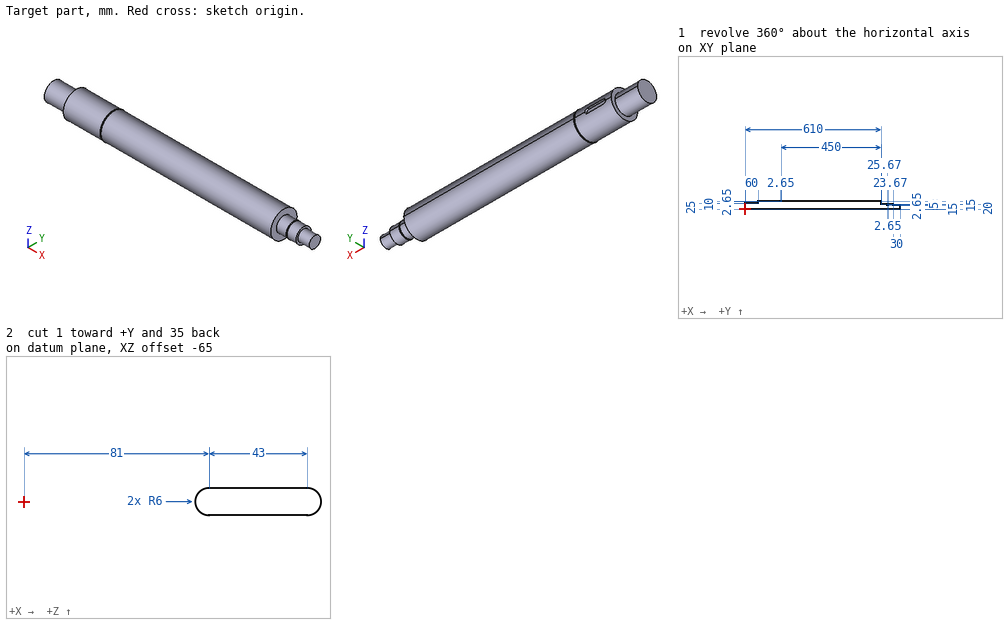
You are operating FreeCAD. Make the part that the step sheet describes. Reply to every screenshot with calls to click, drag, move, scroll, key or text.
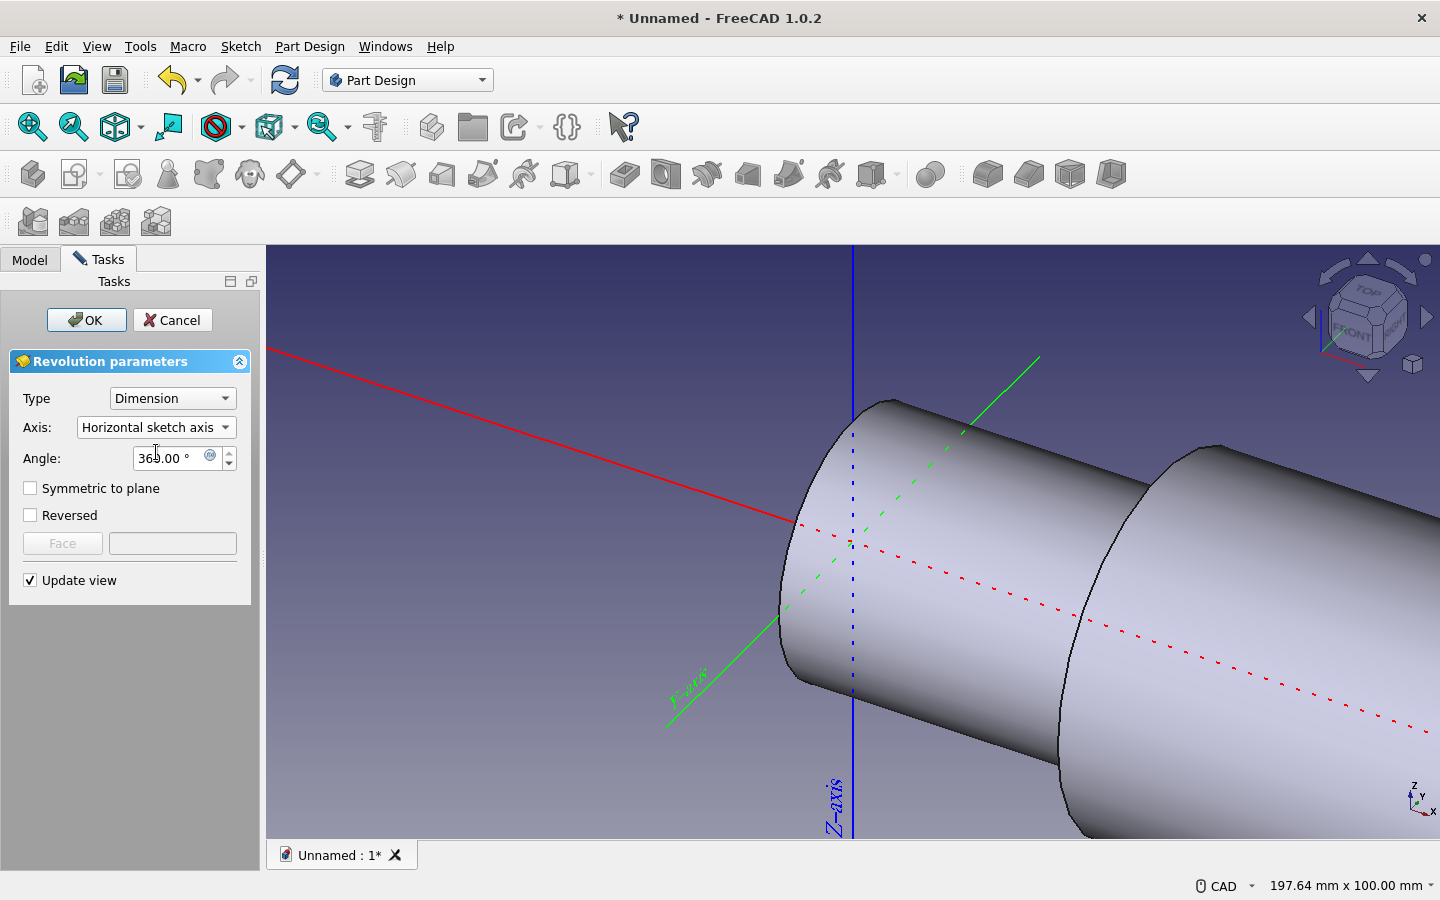
click(87, 320)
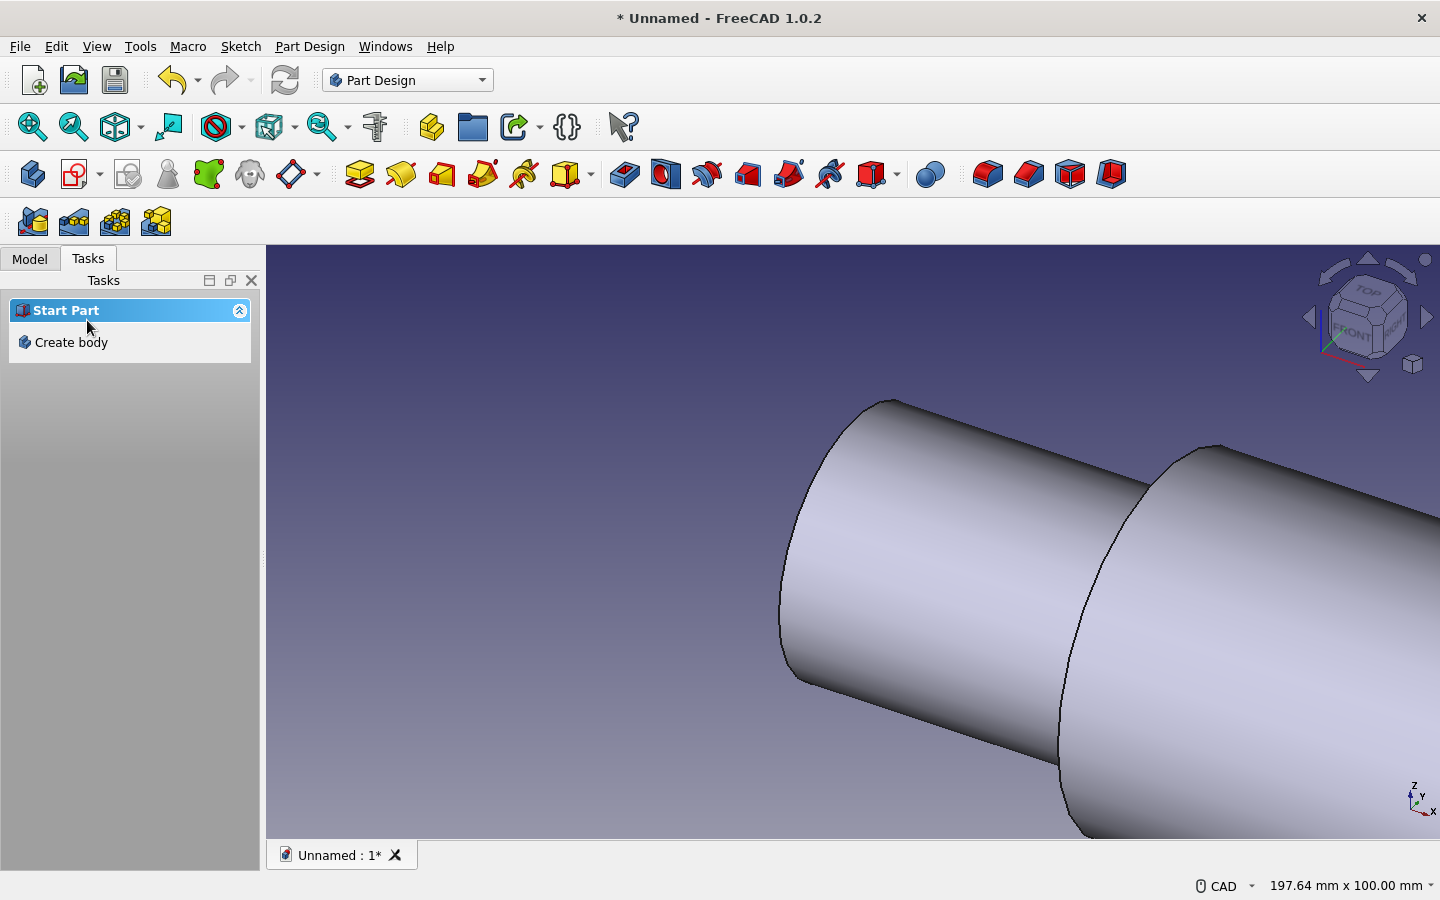
click(33, 128)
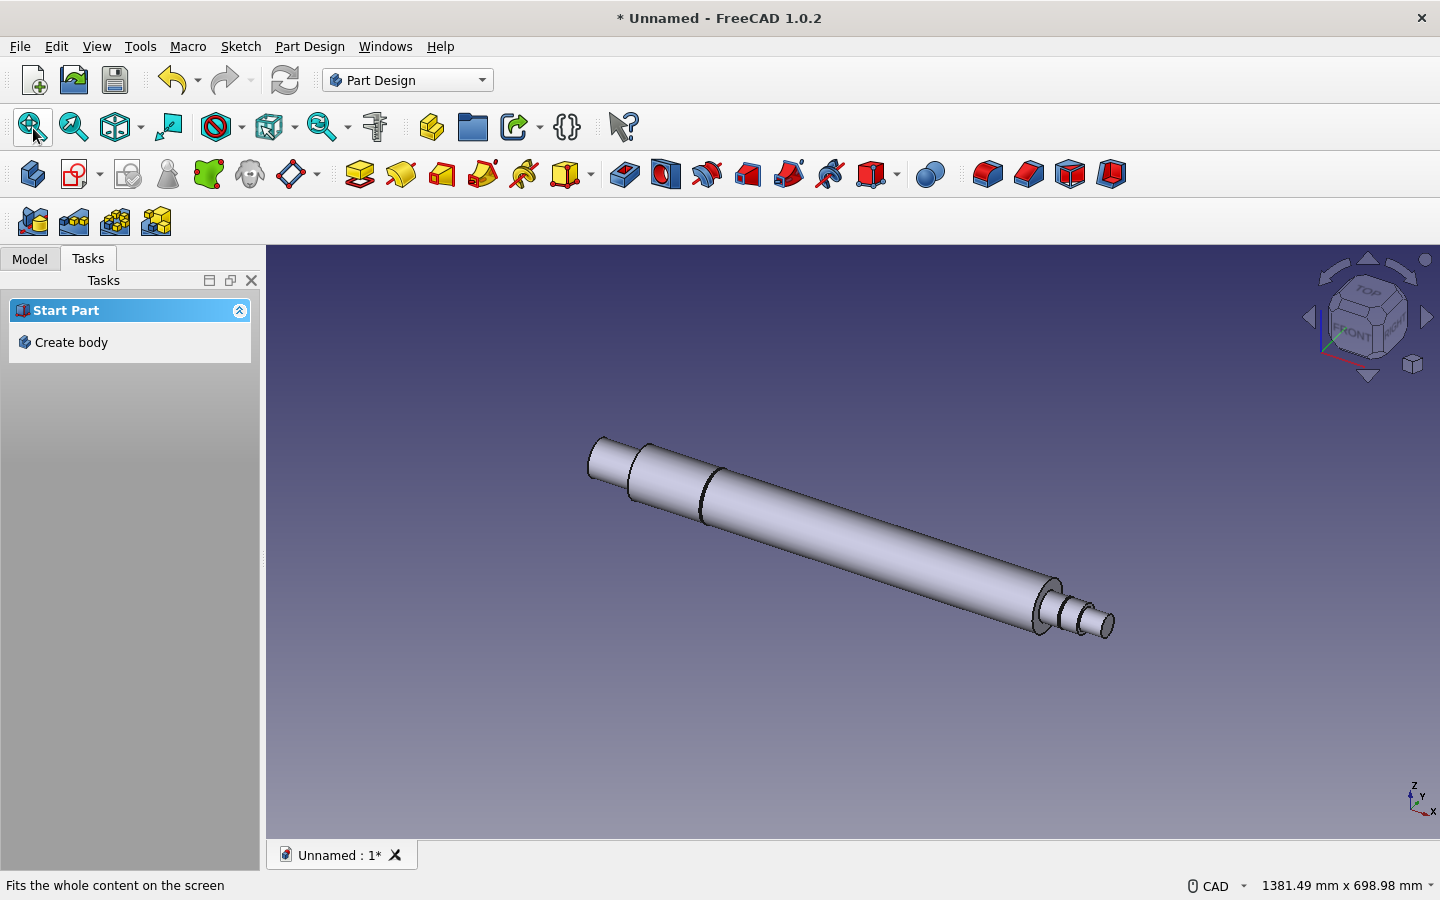
click(30, 258)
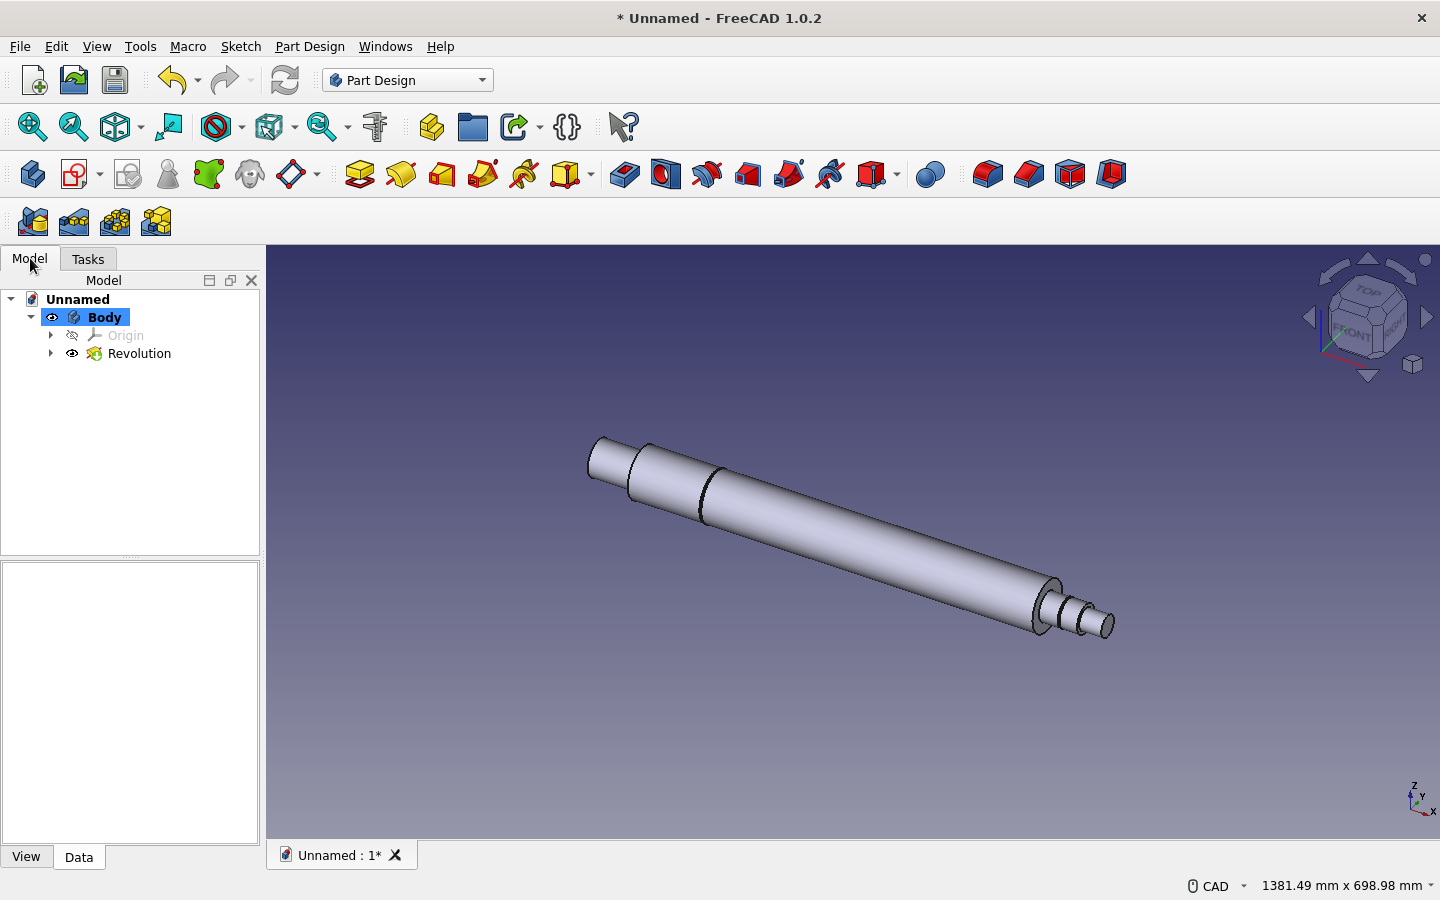
click(51, 335)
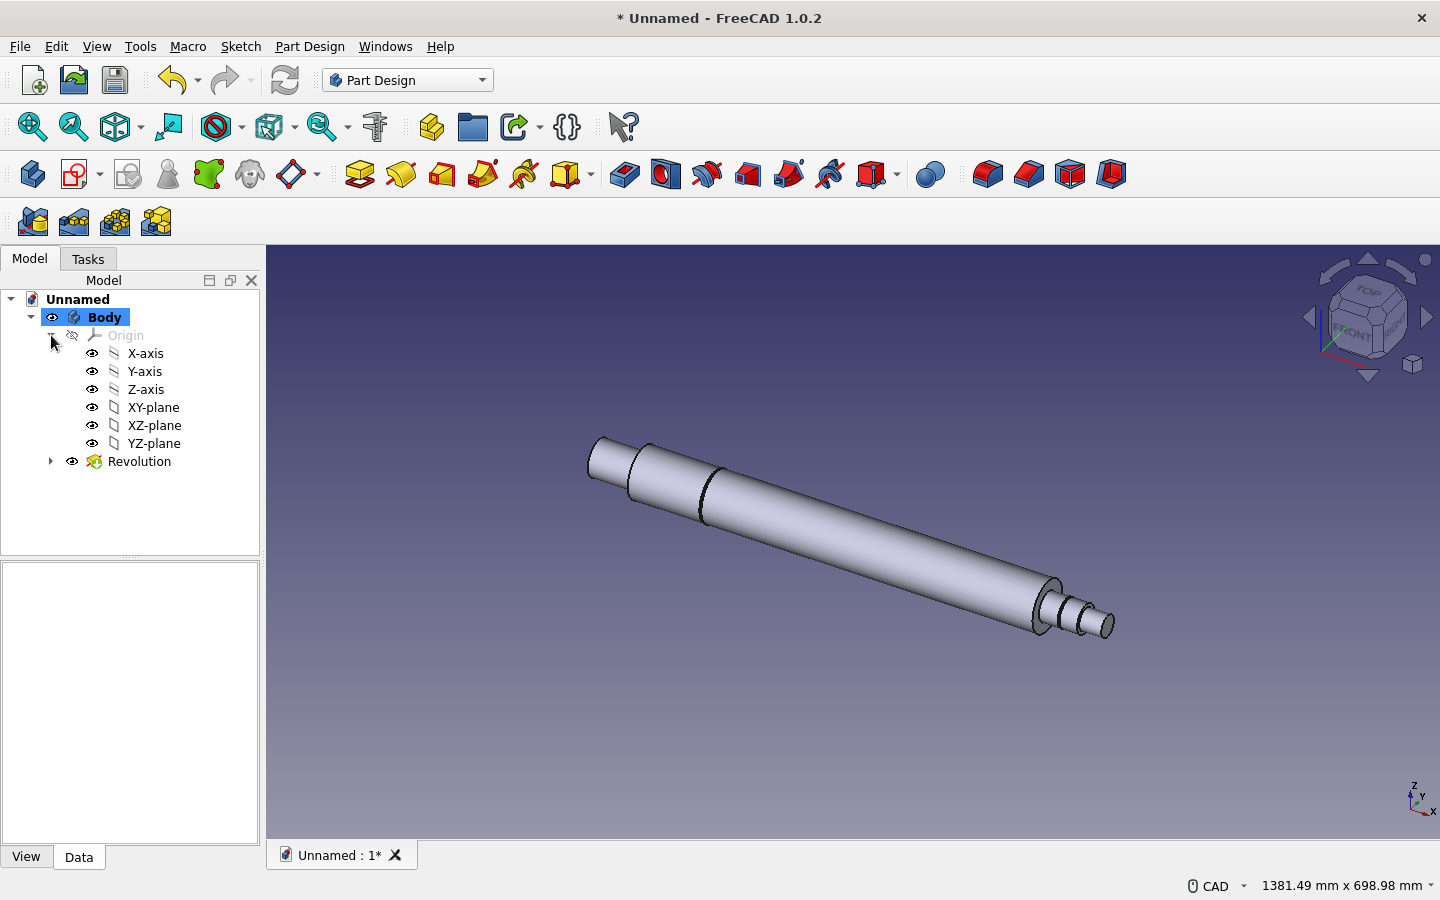
click(137, 425)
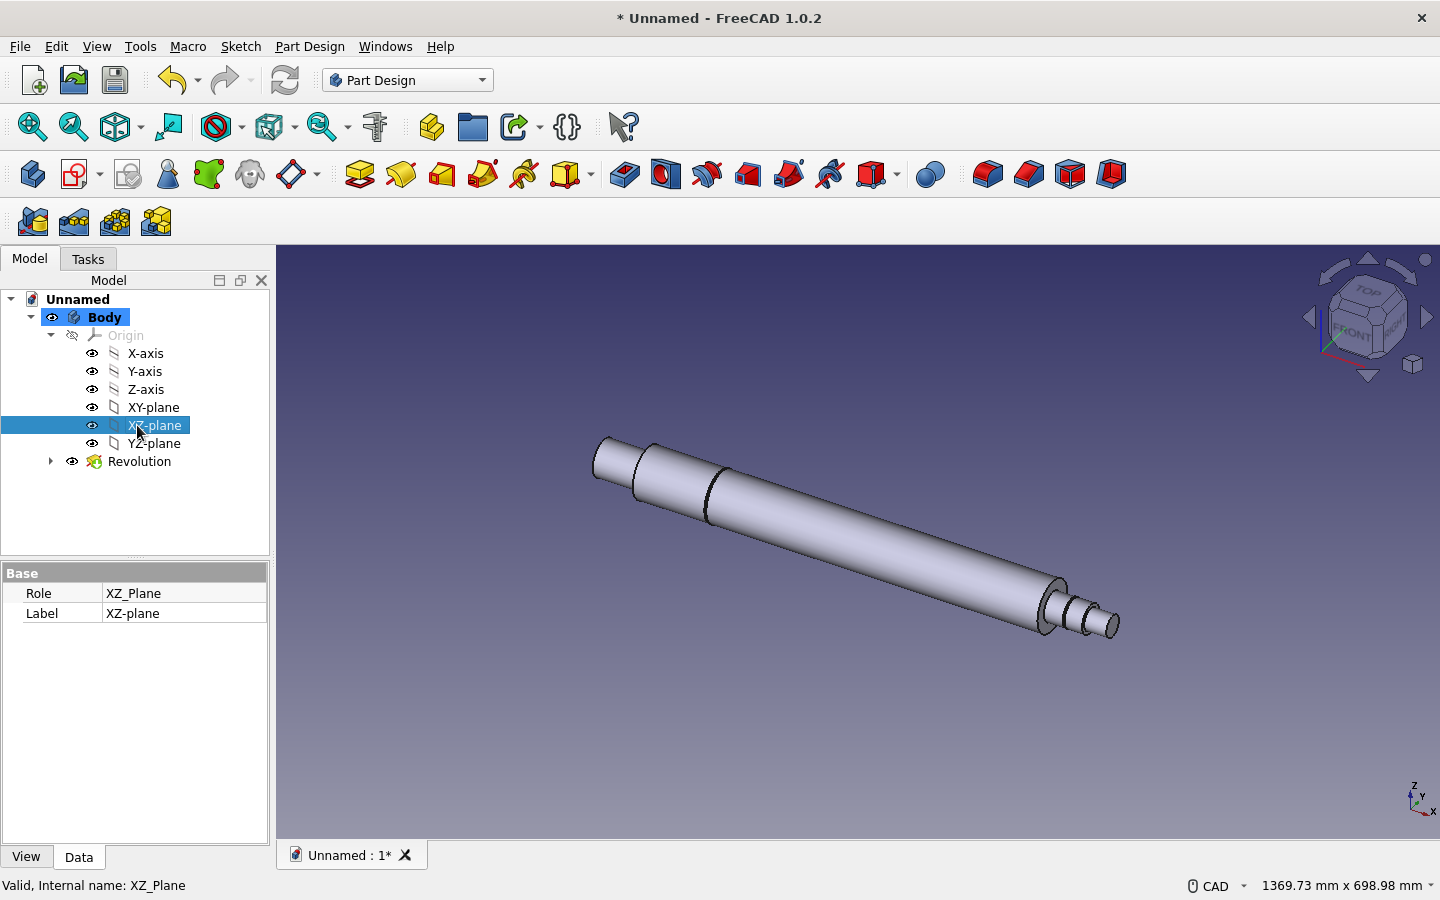
click(290, 174)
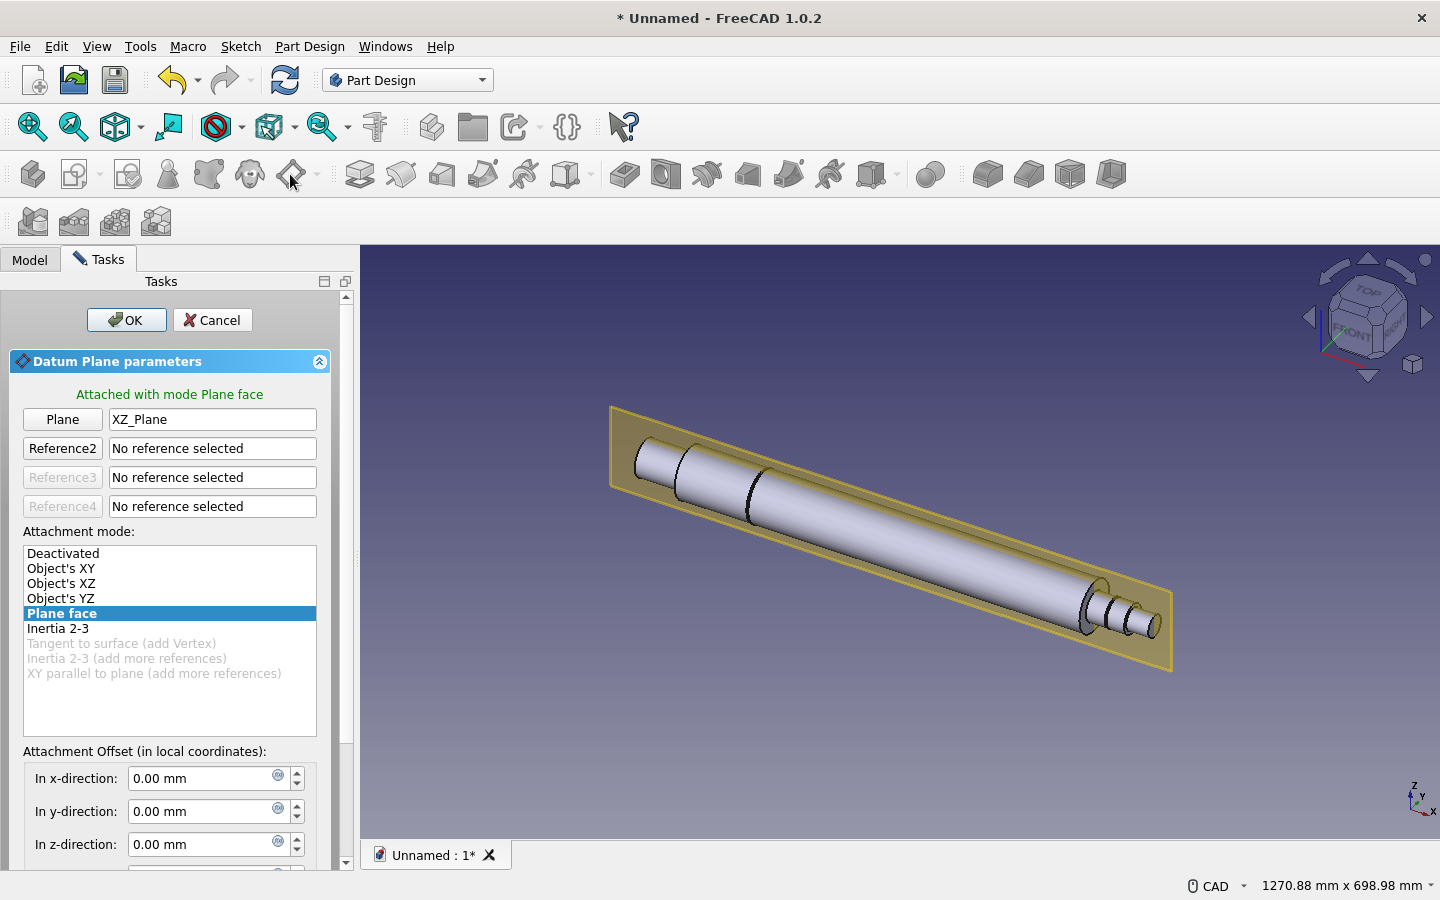
triple_click(210, 844)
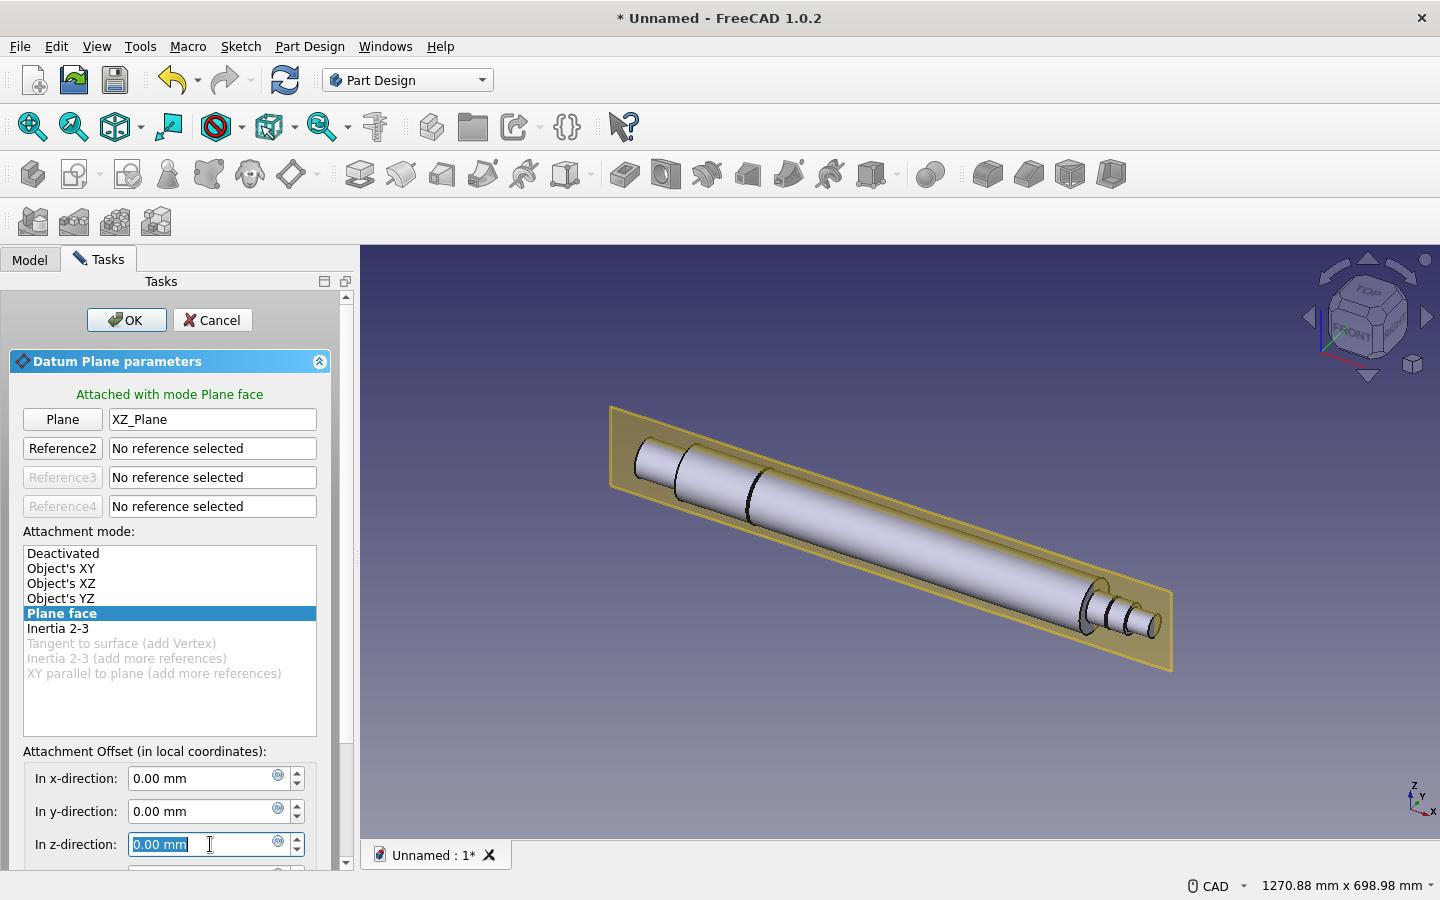
text(-65)
key(Tab)